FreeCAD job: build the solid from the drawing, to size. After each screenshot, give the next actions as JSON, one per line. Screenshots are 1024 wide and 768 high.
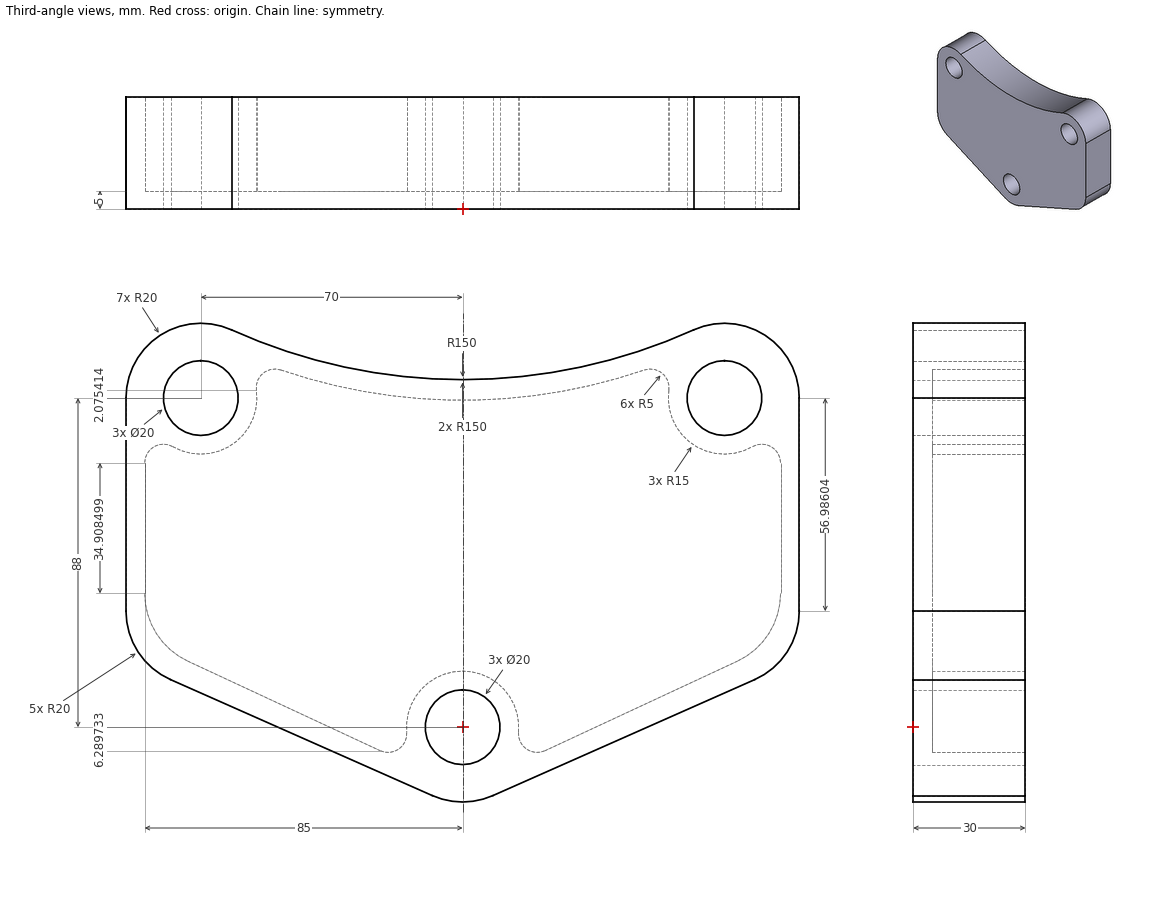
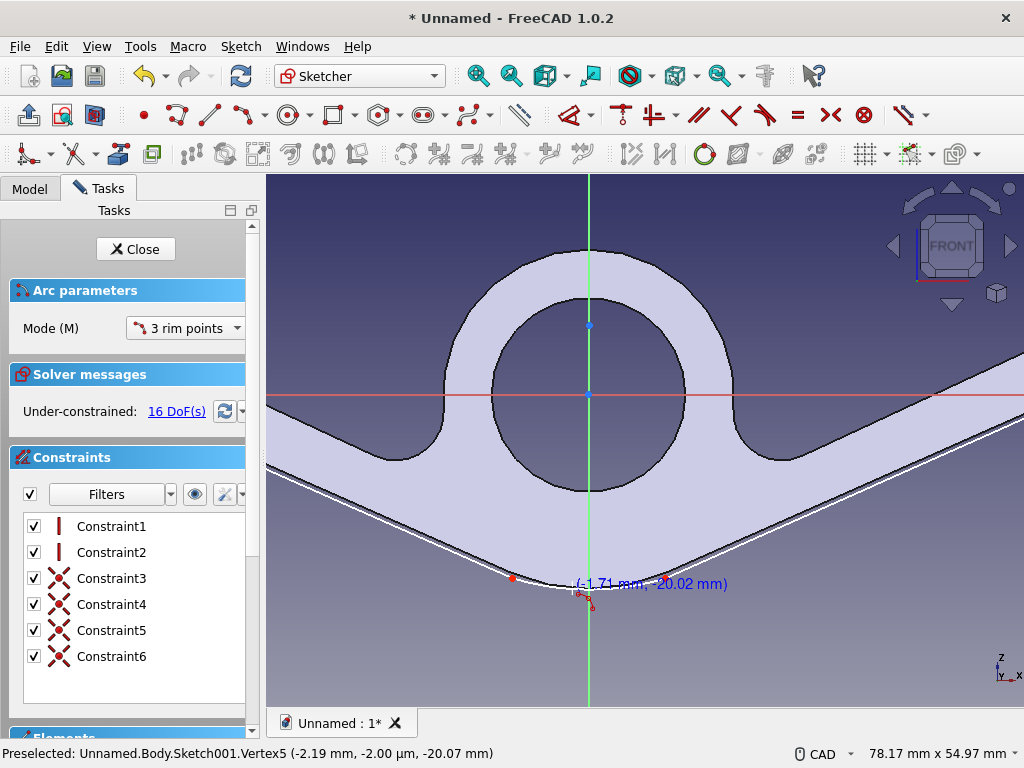
{"action": "scroll", "coordinate": [573, 592], "scroll_direction": "down", "scroll_amount": 7}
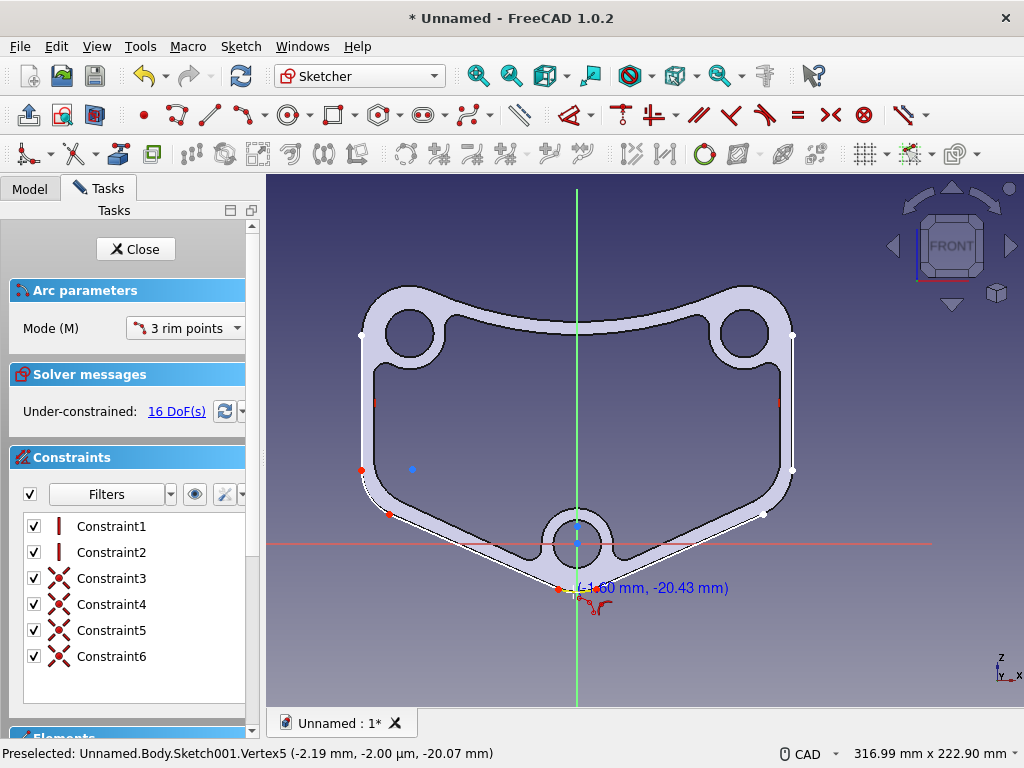
{"action": "left_click", "coordinate": [764, 515]}
{"action": "left_click", "coordinate": [793, 471]}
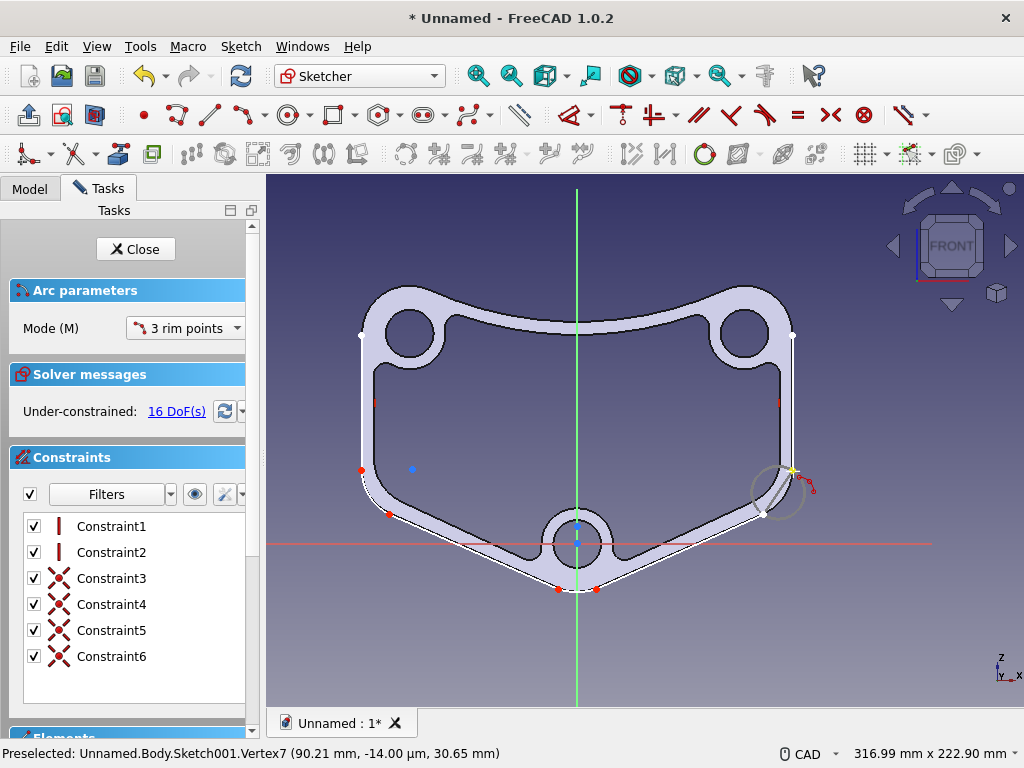
{"action": "scroll", "coordinate": [785, 496], "scroll_direction": "up", "scroll_amount": 4}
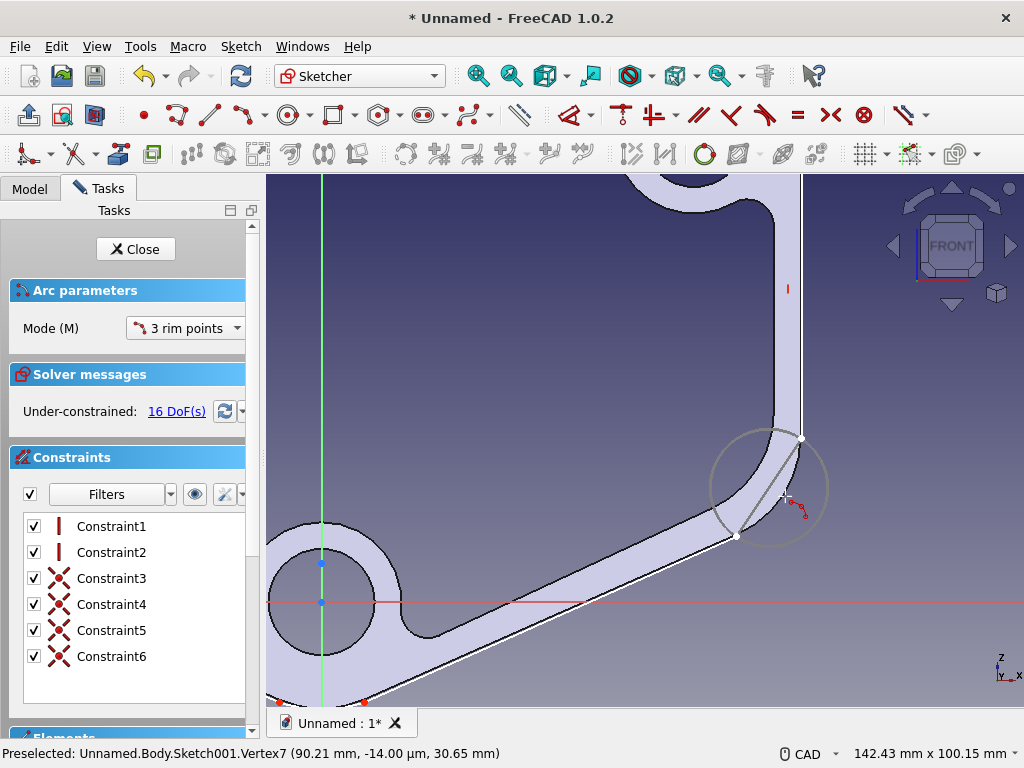
{"action": "left_click", "coordinate": [783, 495]}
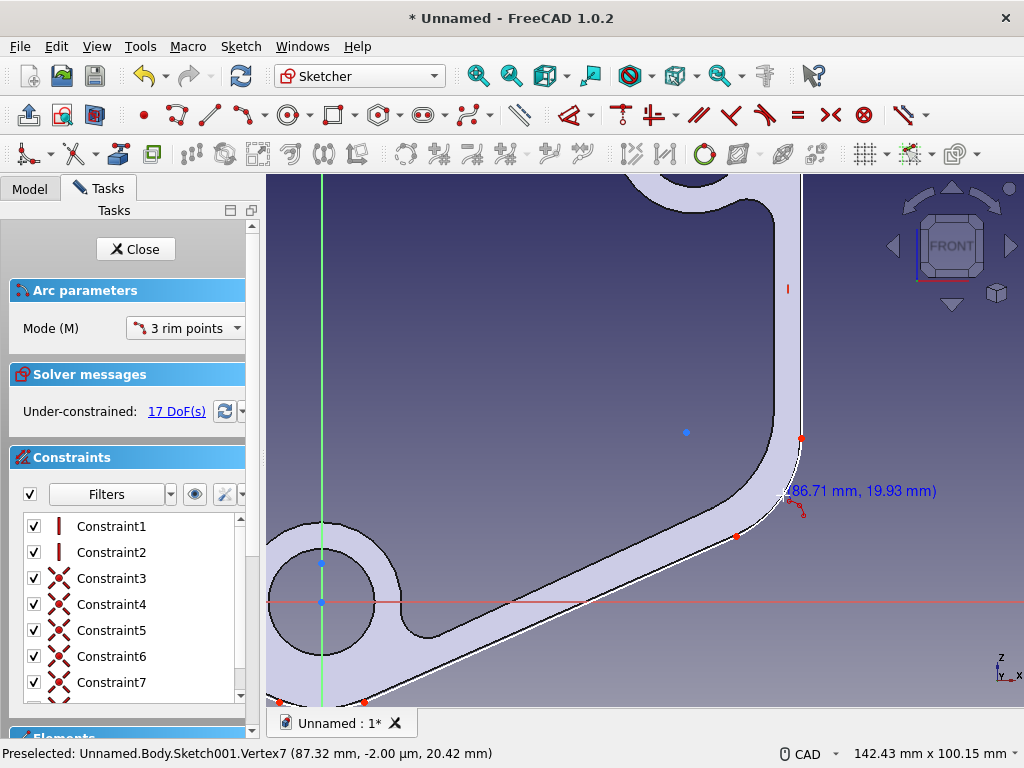
{"action": "scroll", "coordinate": [785, 496], "scroll_direction": "down", "scroll_amount": 4}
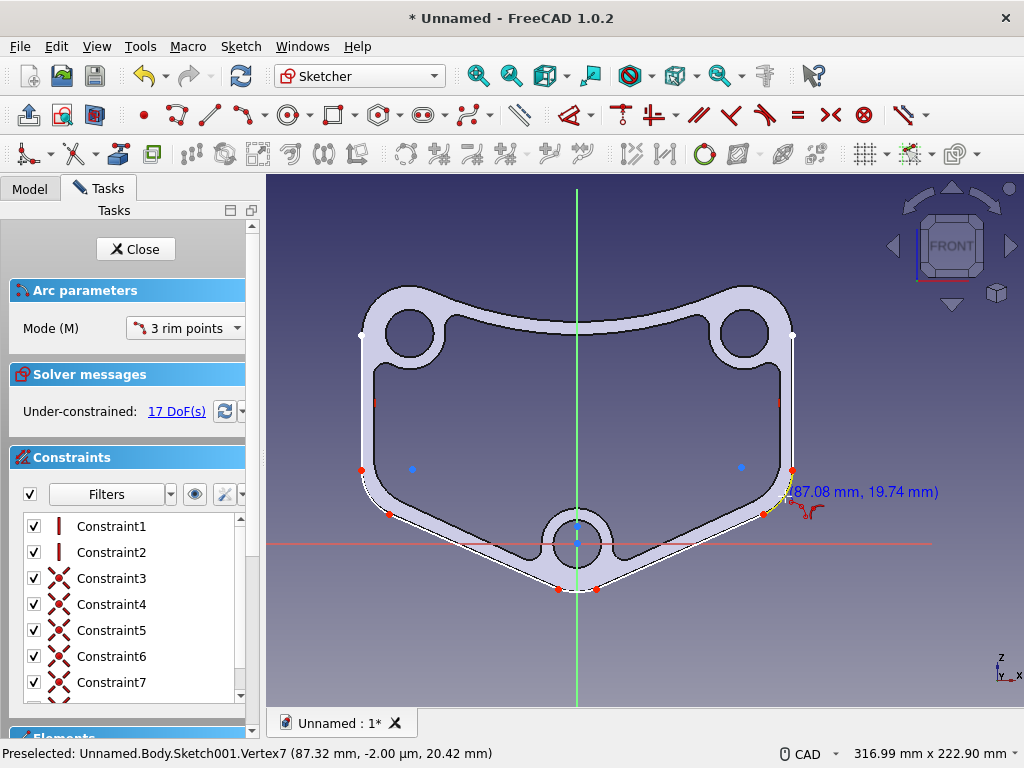
{"action": "left_click", "coordinate": [793, 335]}
{"action": "left_click", "coordinate": [725, 290]}
{"action": "left_click", "coordinate": [770, 293]}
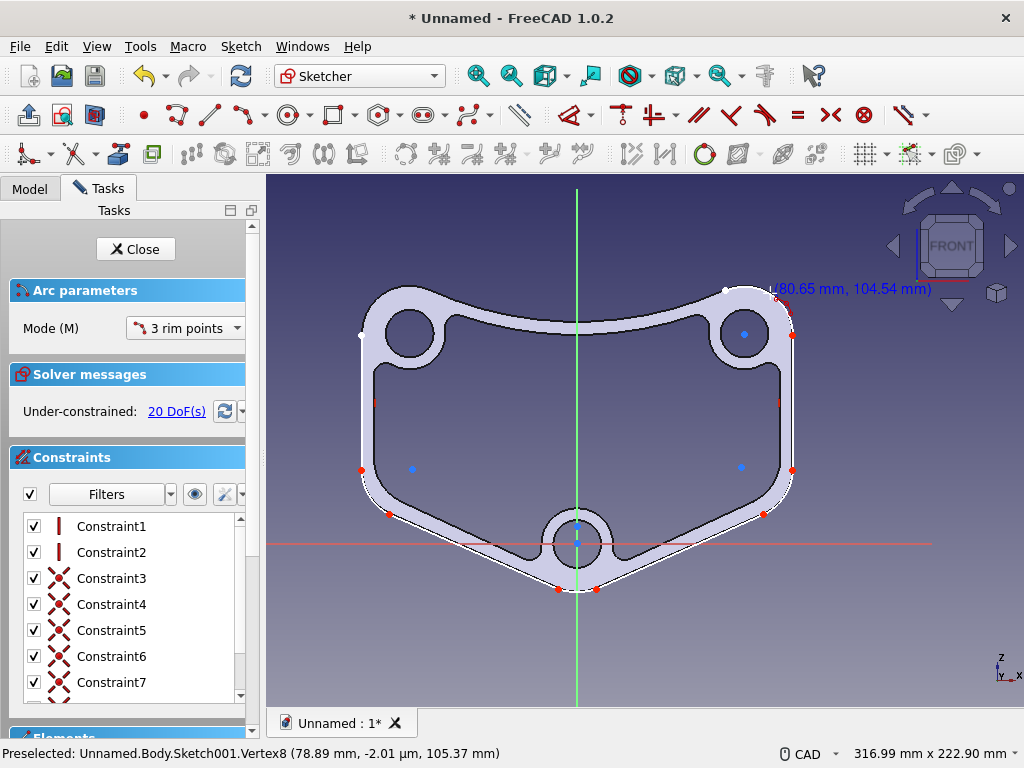
{"action": "left_click", "coordinate": [725, 291]}
{"action": "left_click", "coordinate": [429, 290]}
{"action": "left_click", "coordinate": [547, 321]}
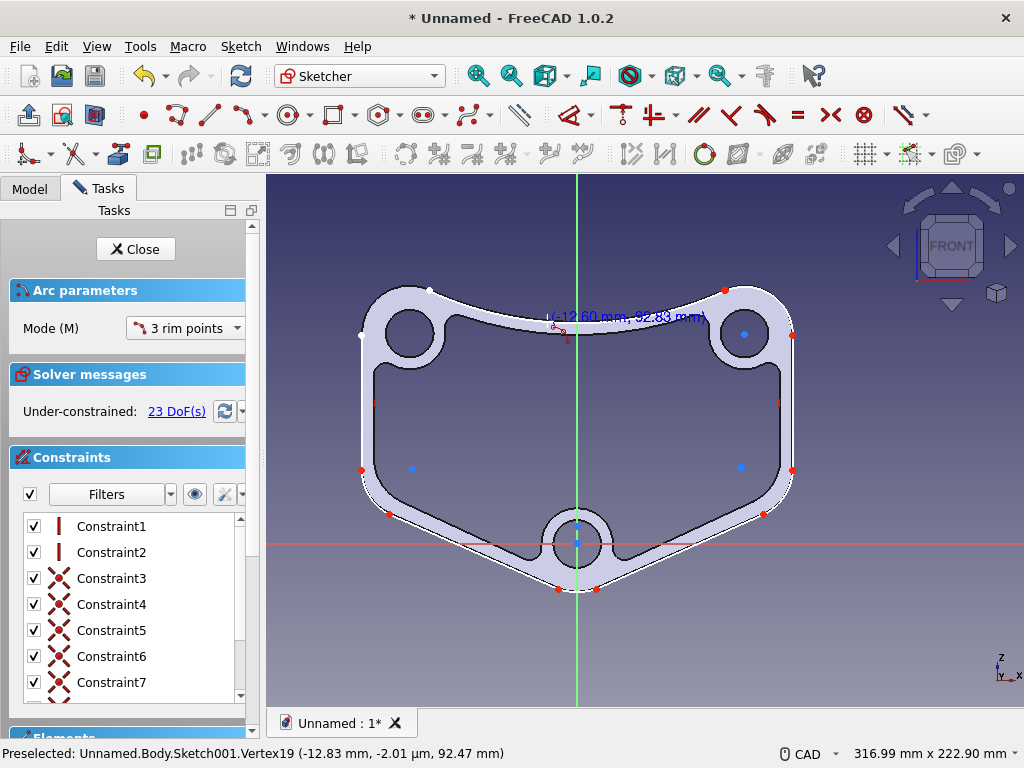
{"action": "left_click", "coordinate": [429, 291]}
{"action": "left_click", "coordinate": [362, 335]}
{"action": "left_click", "coordinate": [384, 293]}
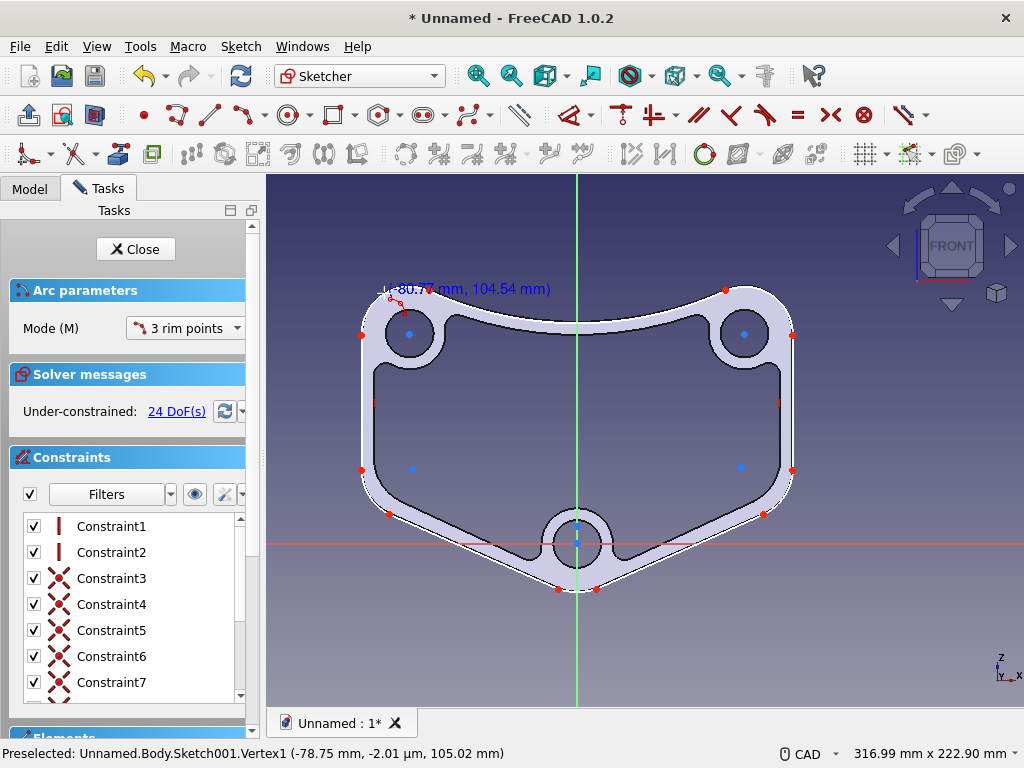
{"action": "left_click", "coordinate": [288, 116]}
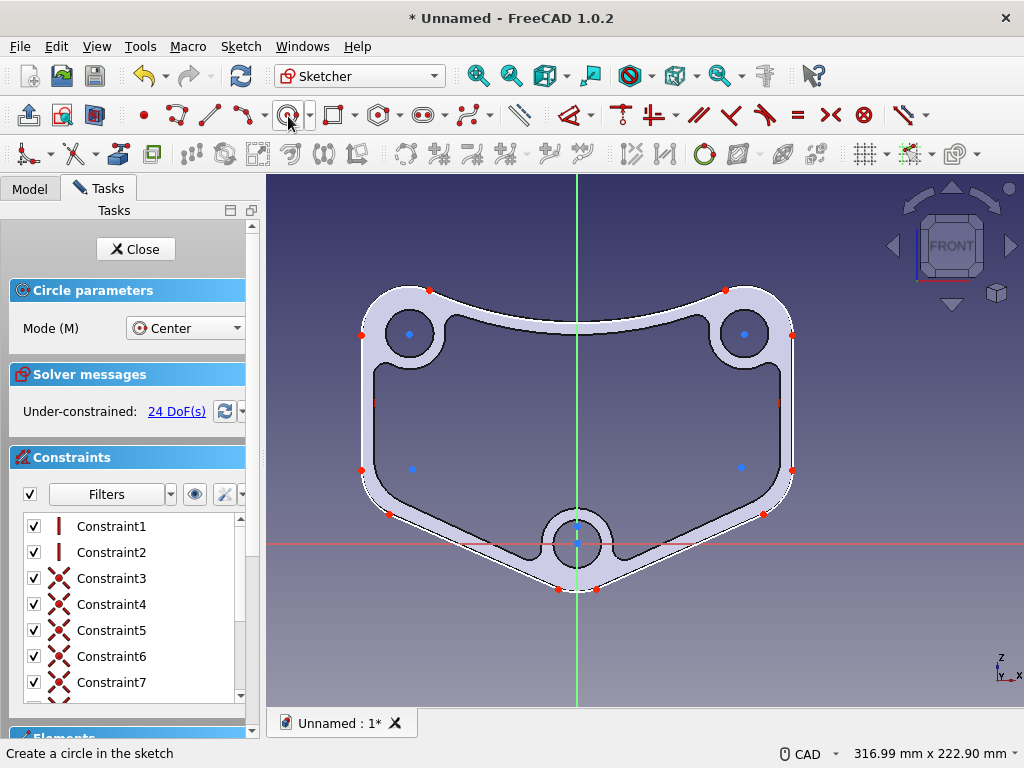
{"action": "left_click", "coordinate": [577, 544]}
{"action": "left_click", "coordinate": [594, 527]}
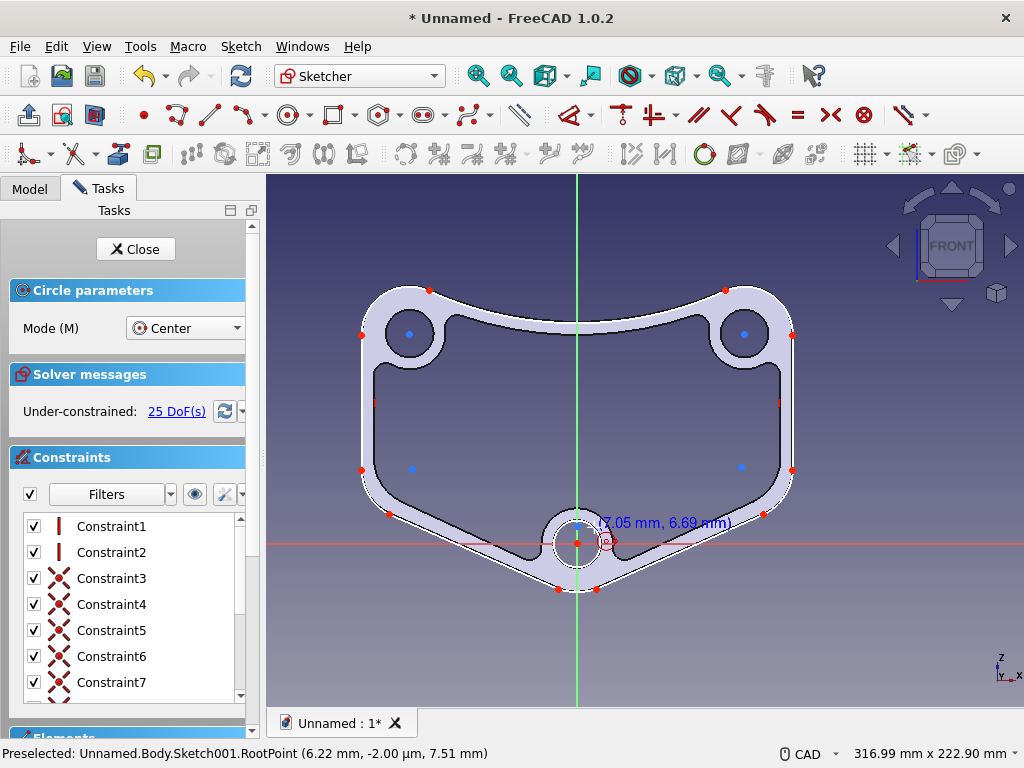
{"action": "left_click", "coordinate": [410, 334]}
{"action": "left_click", "coordinate": [427, 317]}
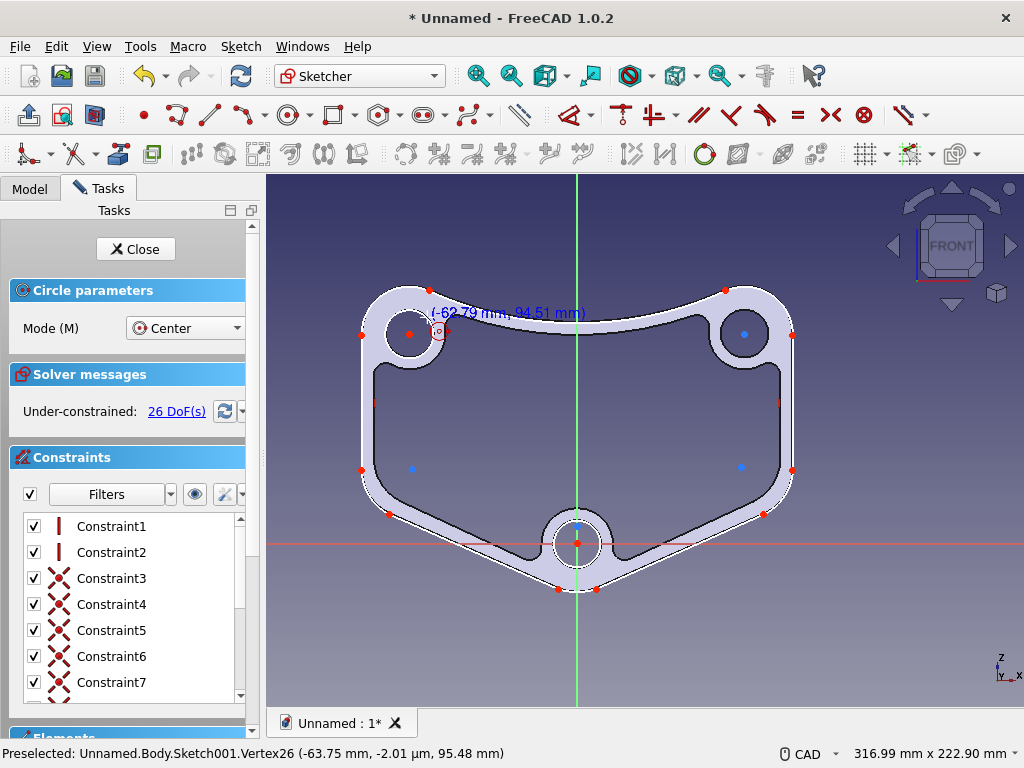
{"action": "left_click", "coordinate": [745, 334]}
{"action": "left_click", "coordinate": [761, 317]}
{"action": "key", "text": "Escape"}